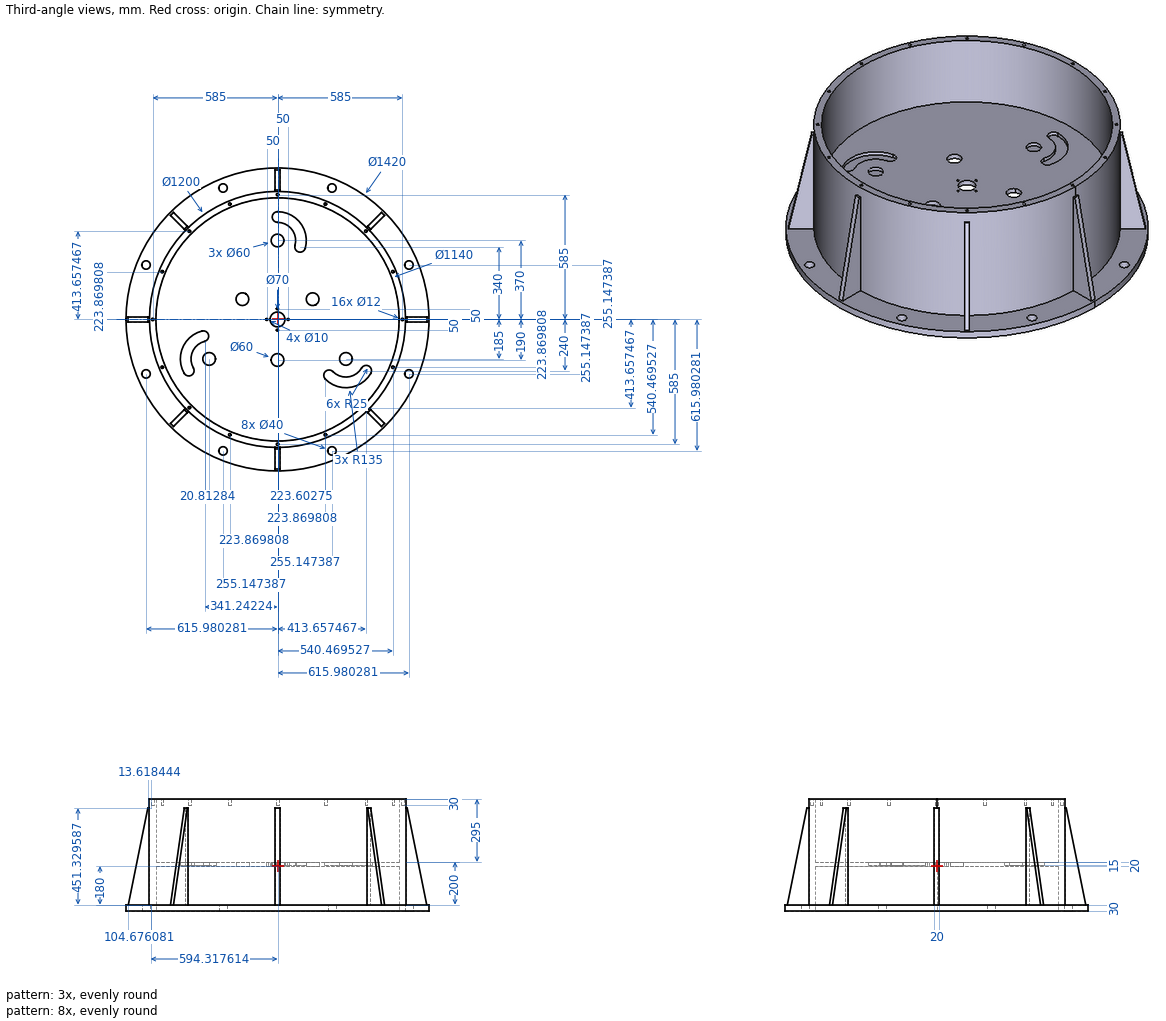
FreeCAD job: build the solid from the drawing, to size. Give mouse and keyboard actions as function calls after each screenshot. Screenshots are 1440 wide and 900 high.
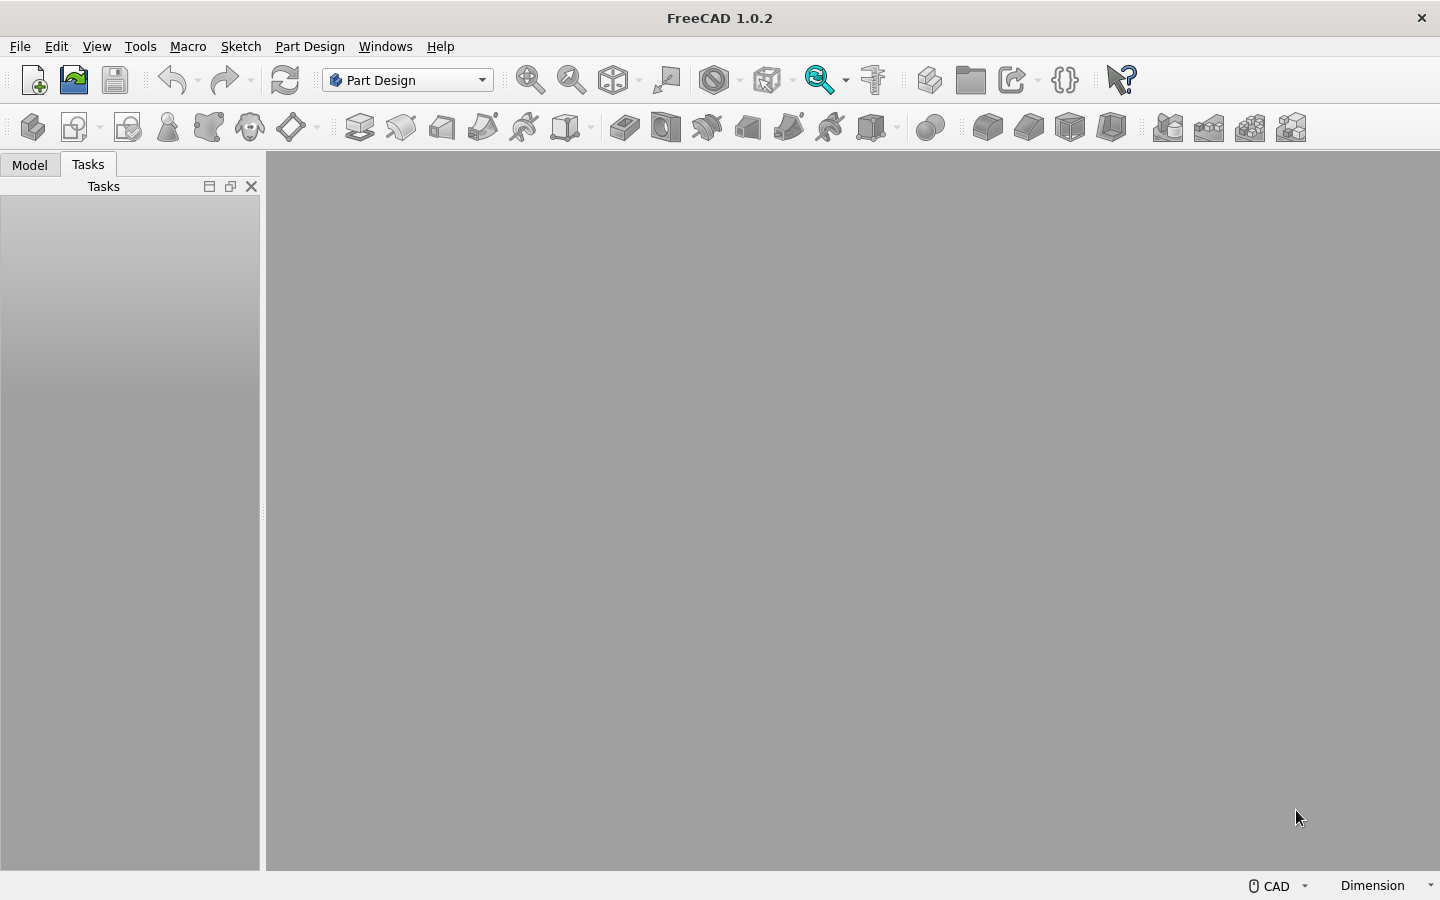
key(ctrl+n)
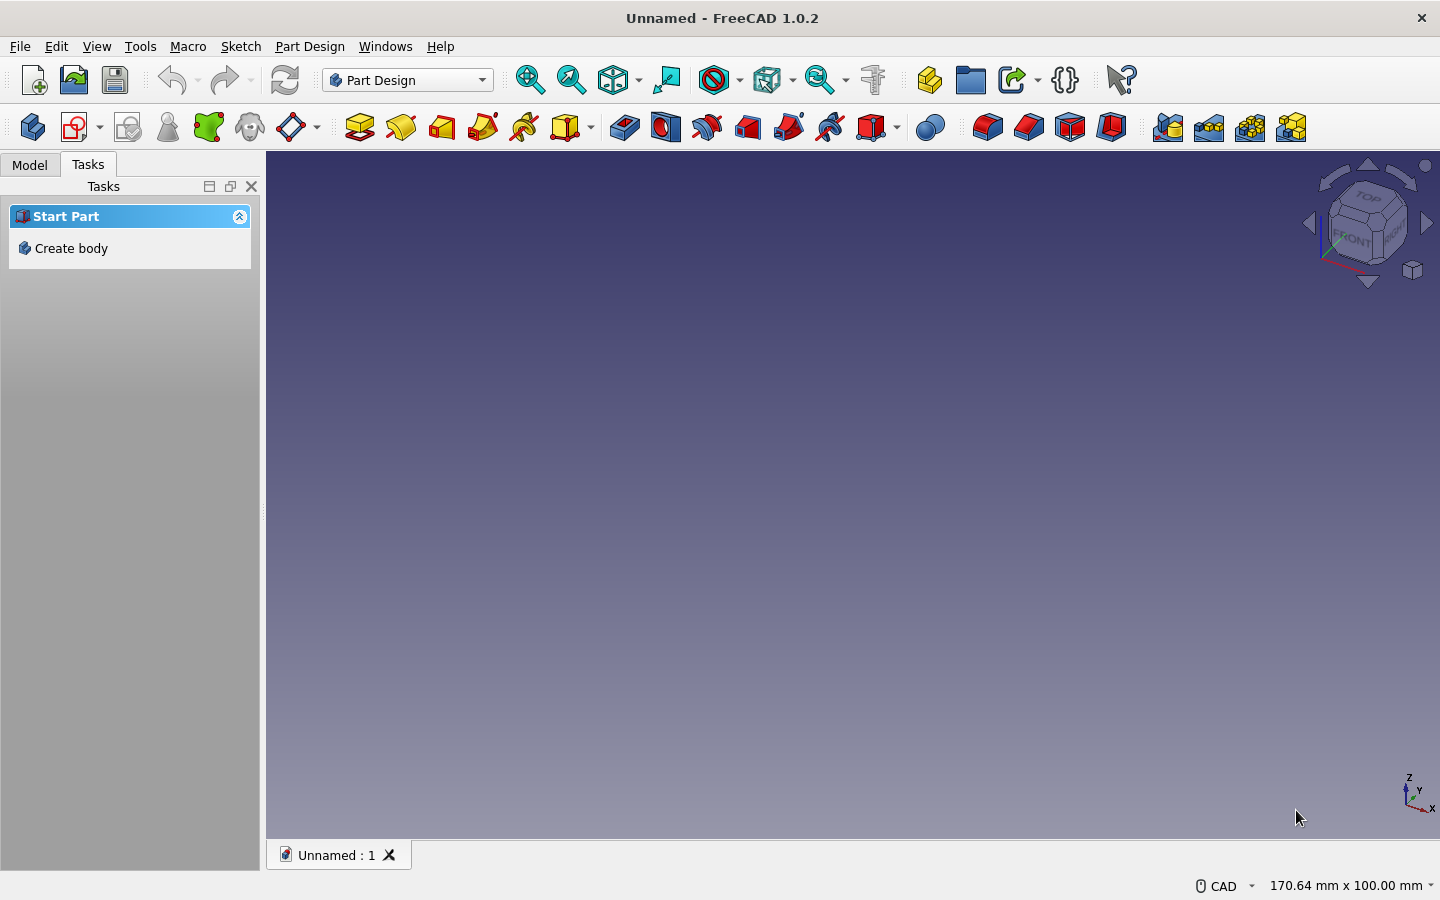
click(74, 128)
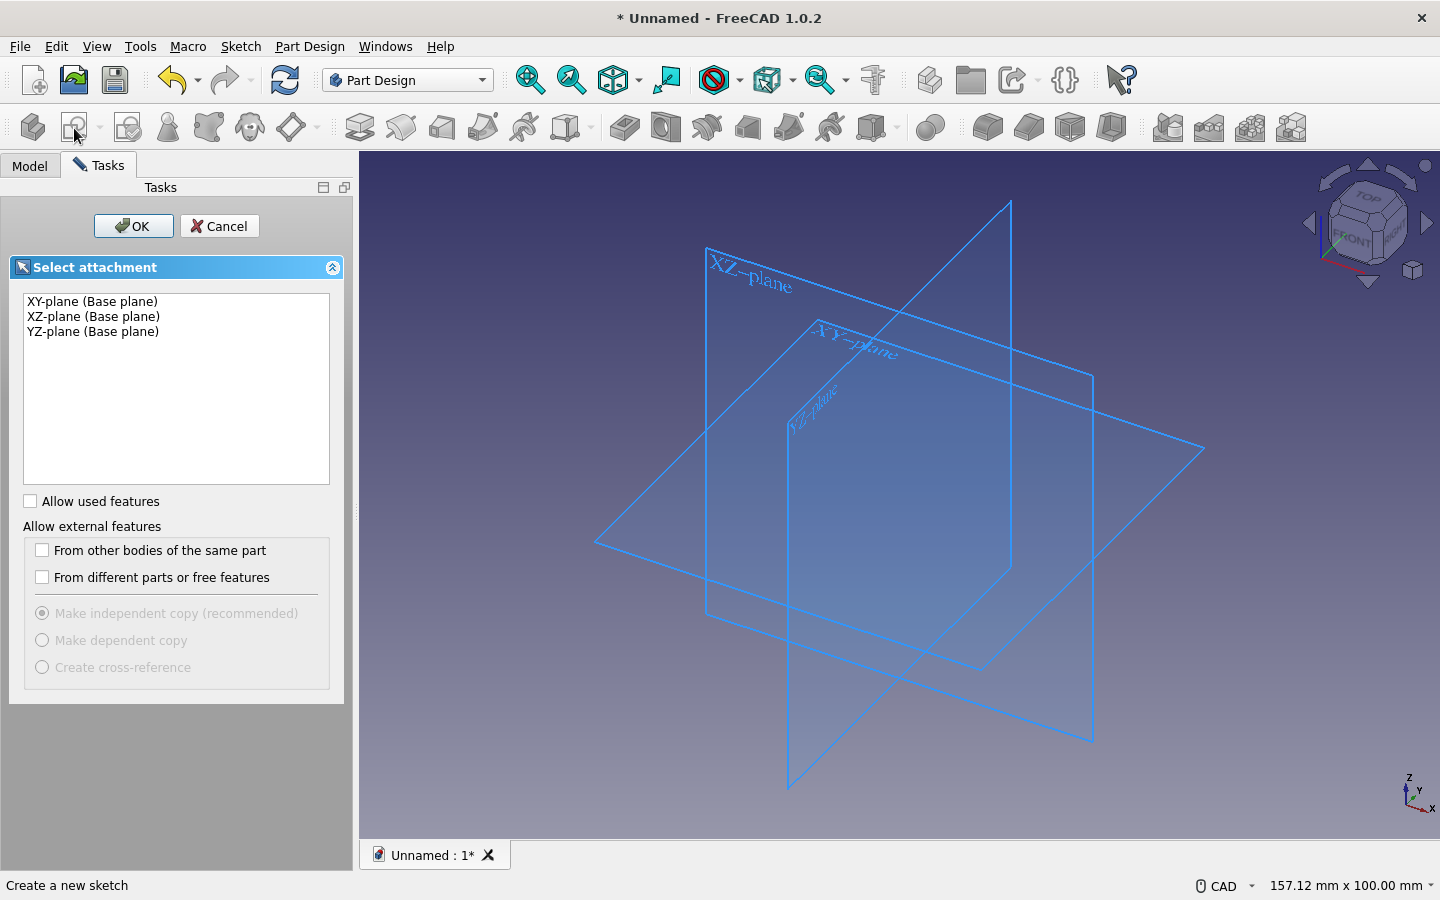
click(84, 302)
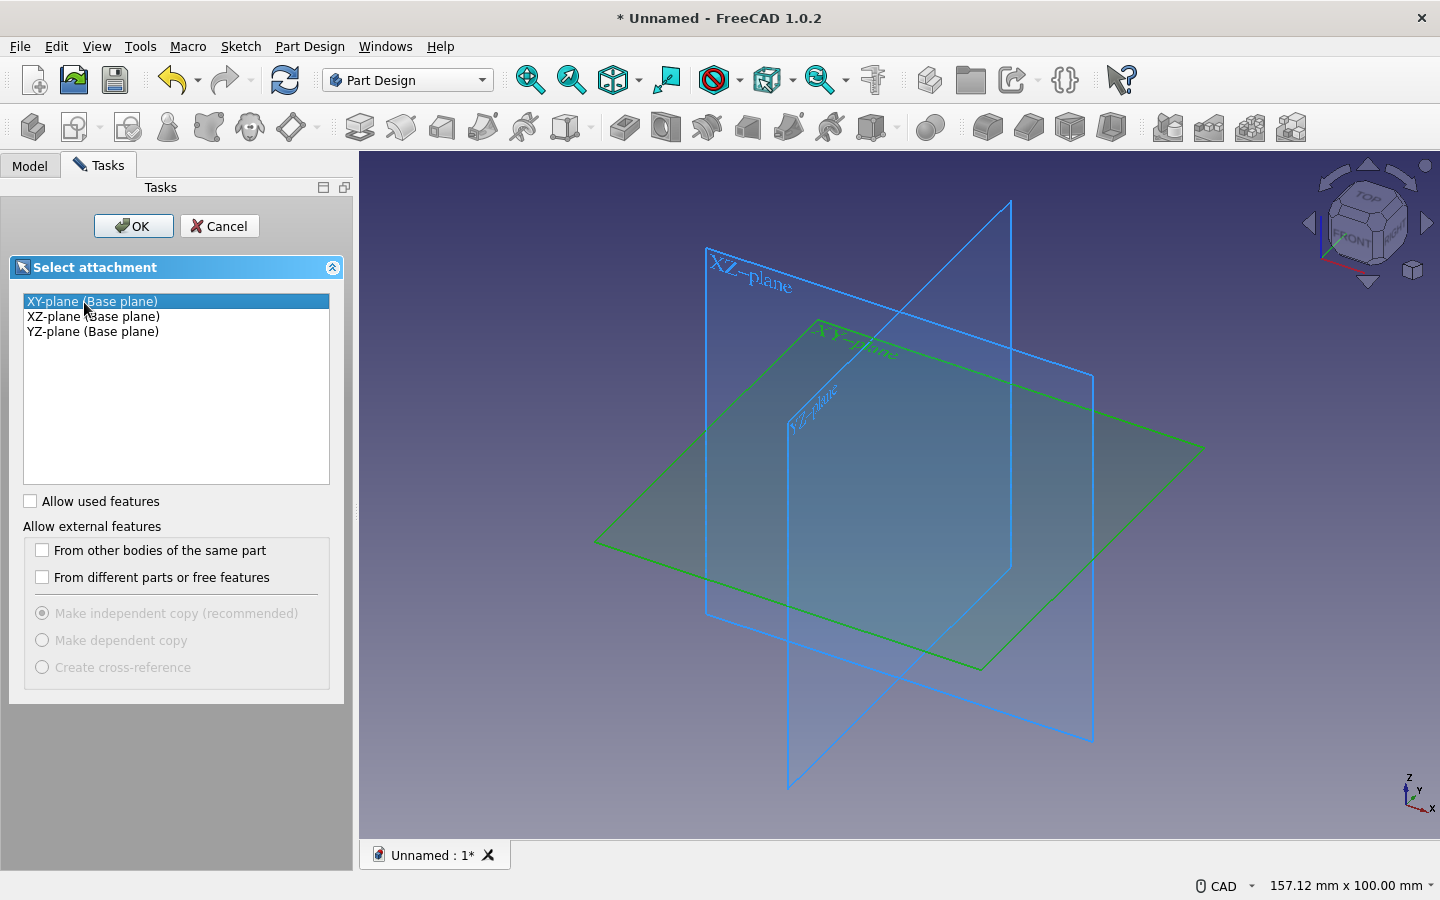
click(134, 226)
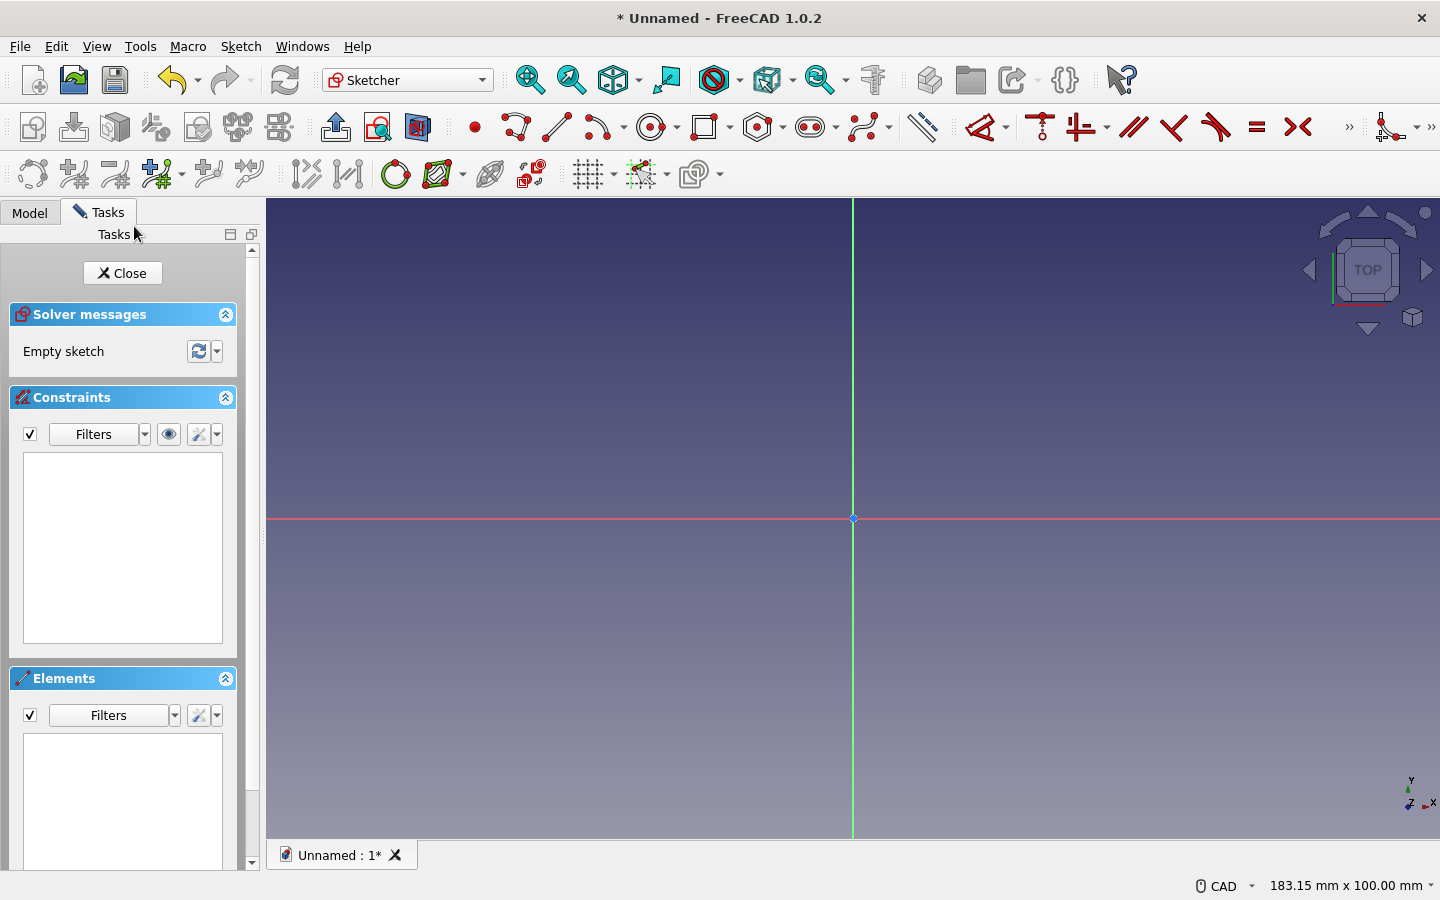
scroll(781, 518, down, 15)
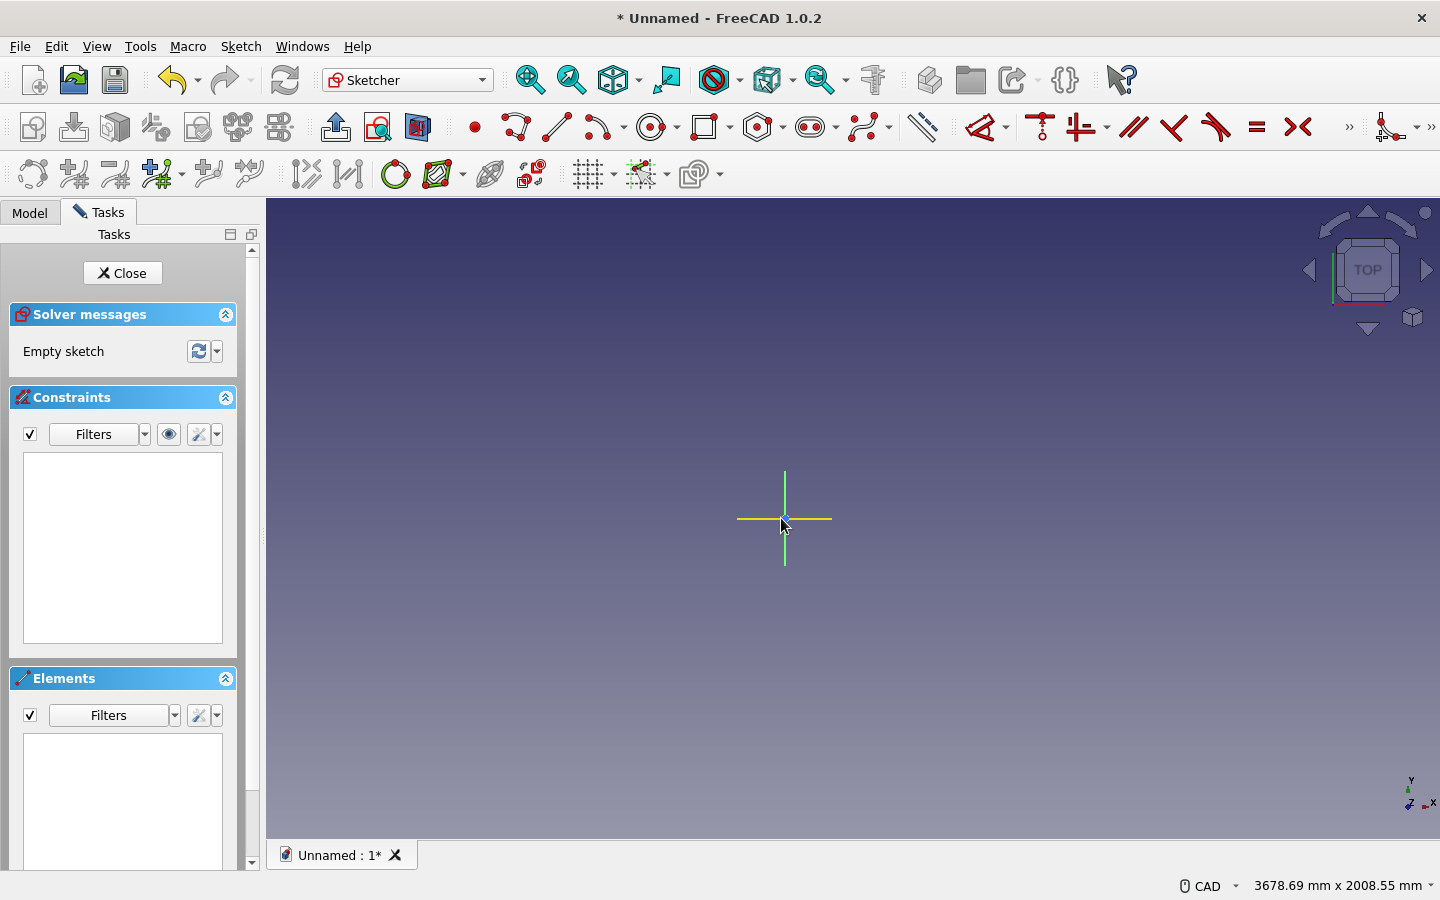
click(650, 128)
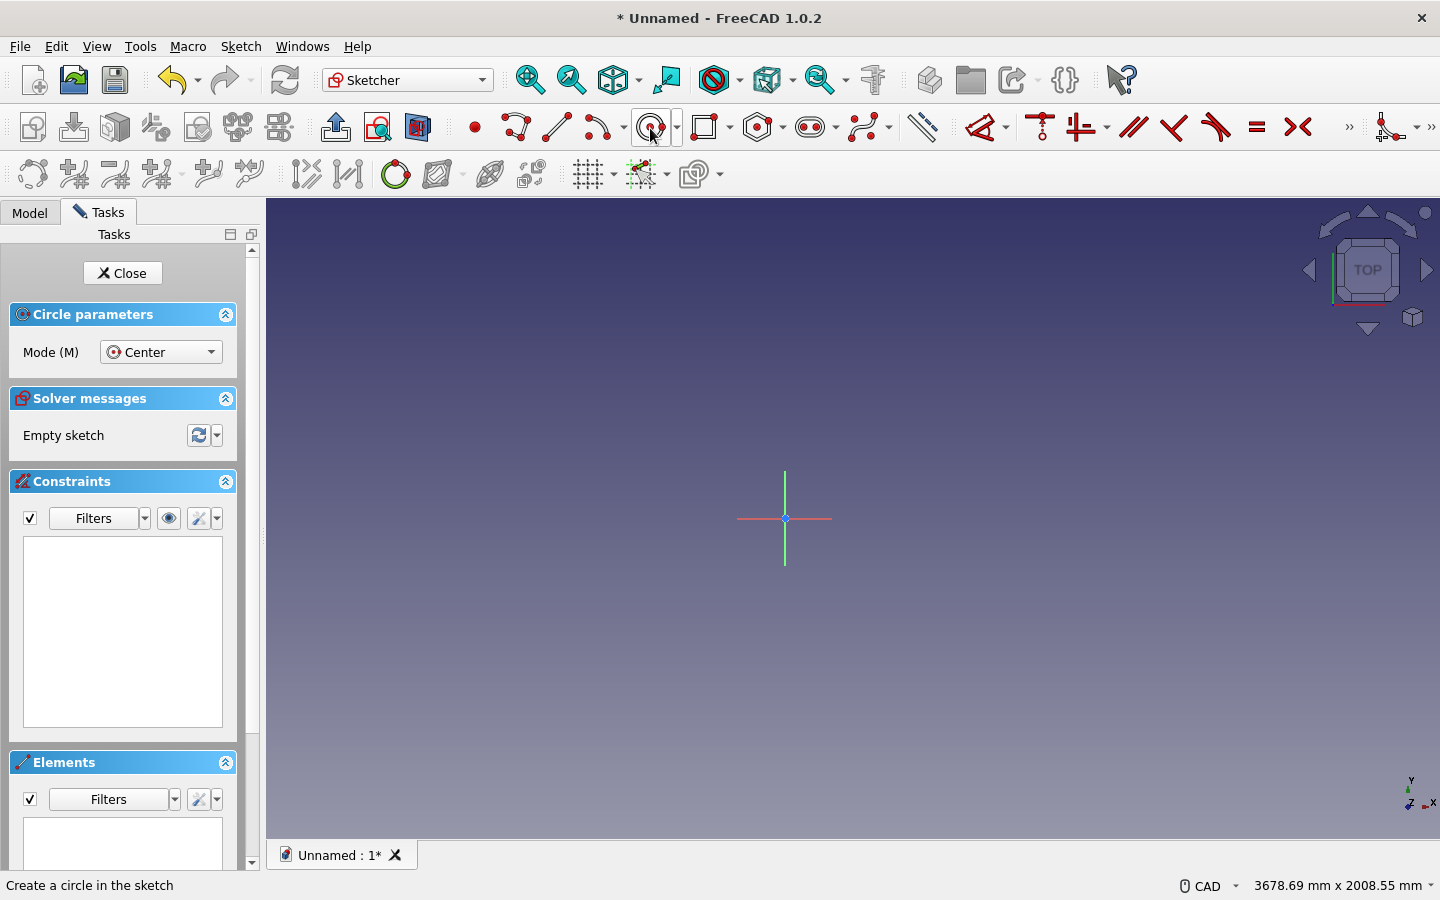
click(785, 518)
move(920, 383)